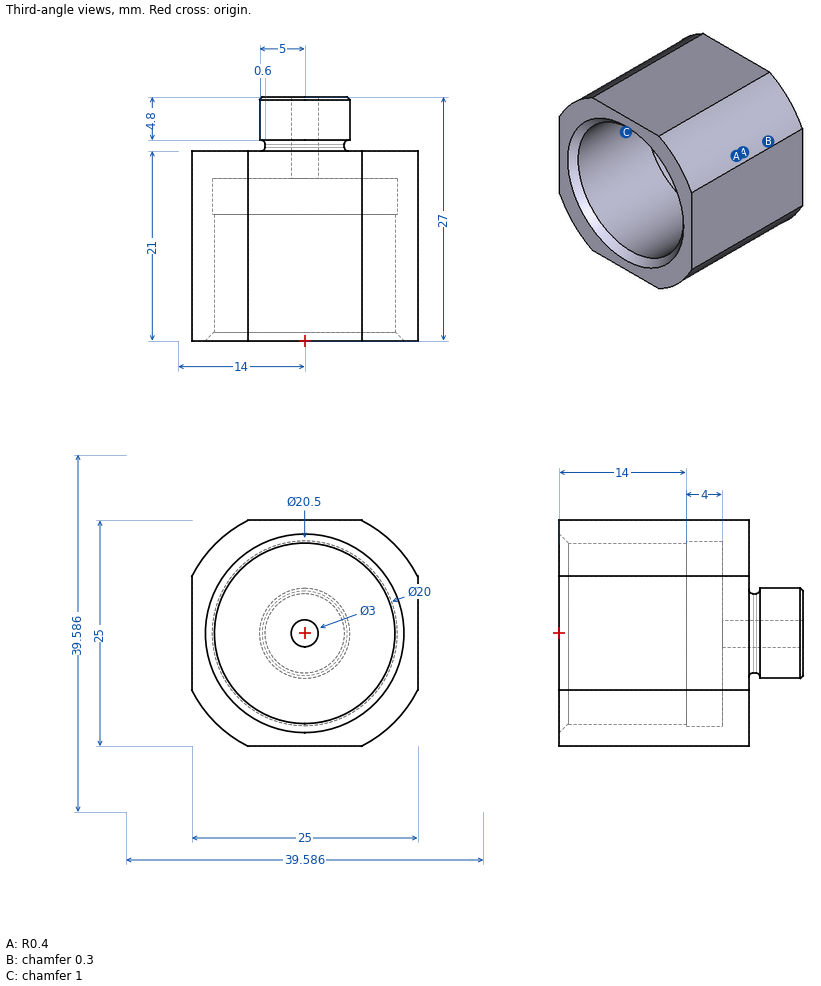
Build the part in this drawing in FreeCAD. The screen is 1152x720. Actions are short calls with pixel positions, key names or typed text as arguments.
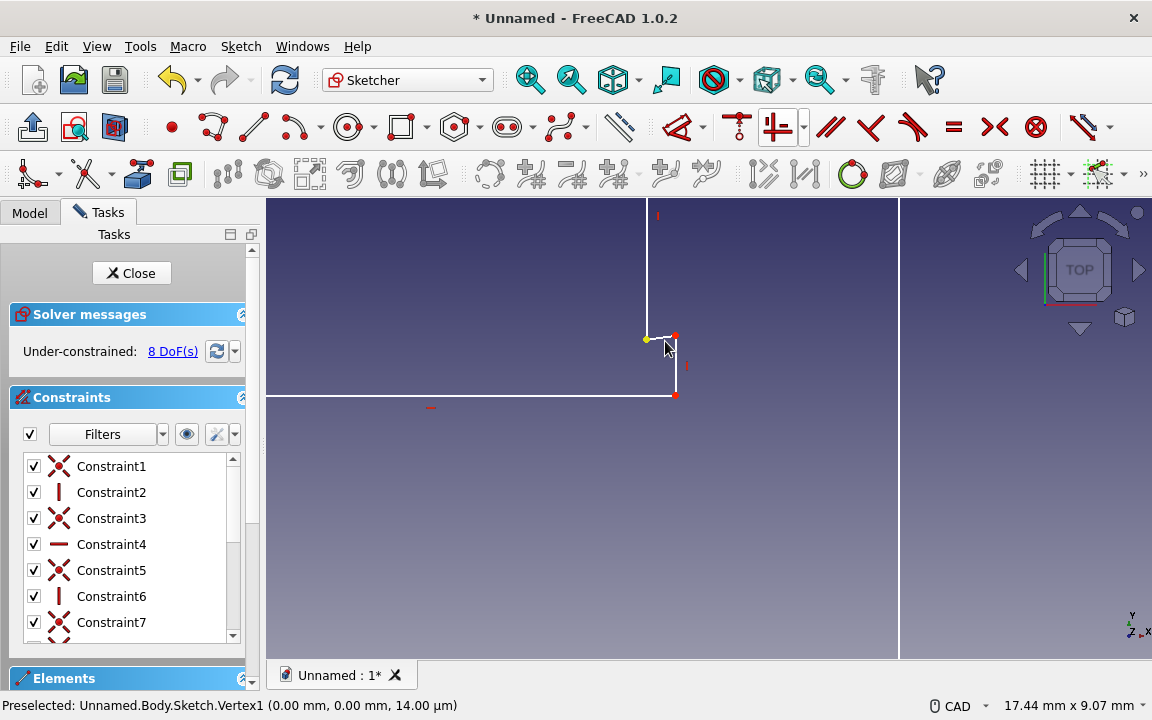
click(661, 338)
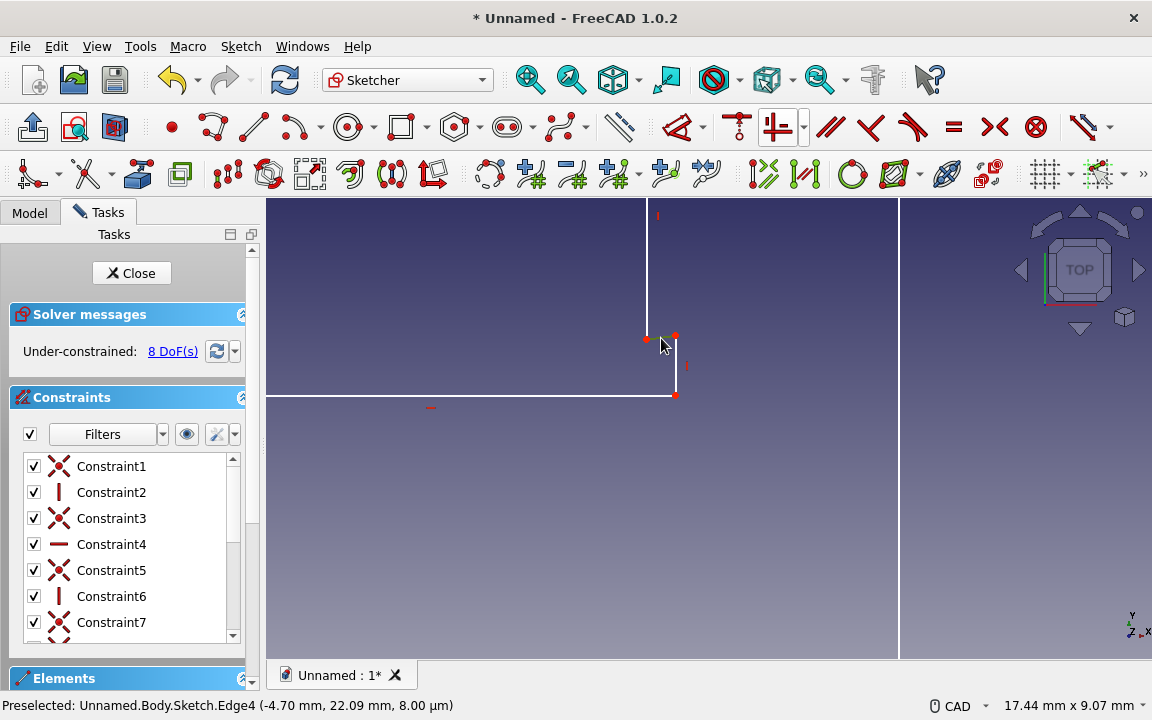
key(h)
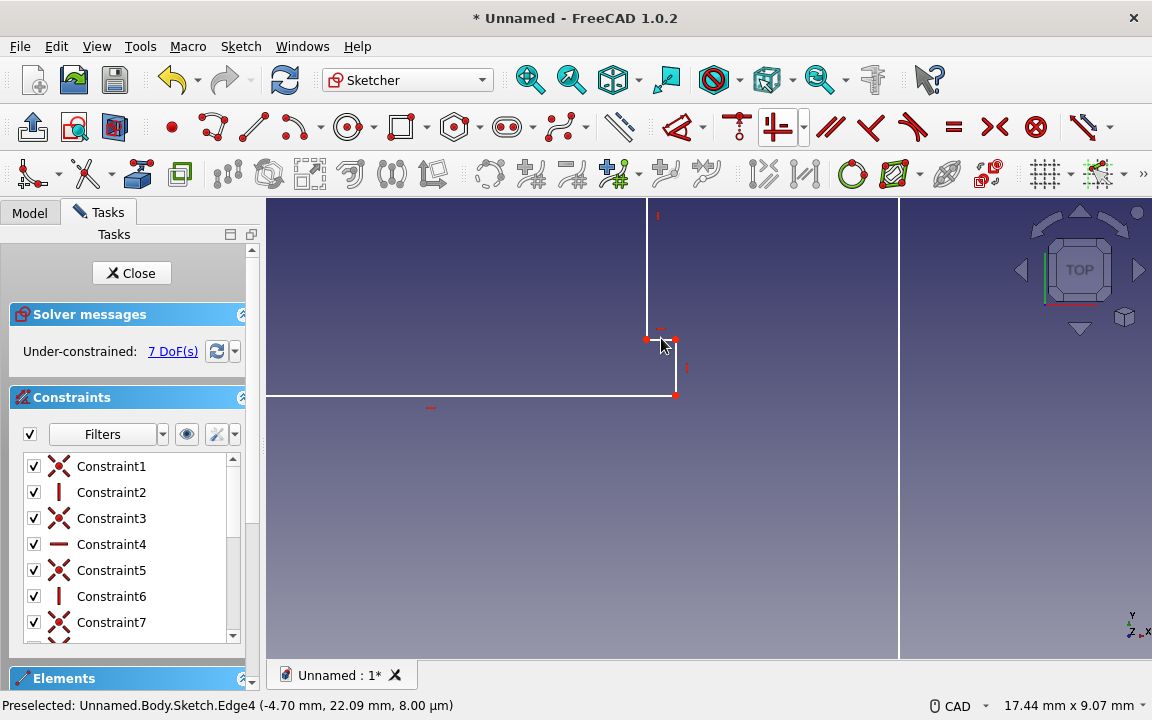
scroll(665, 341, down, 8)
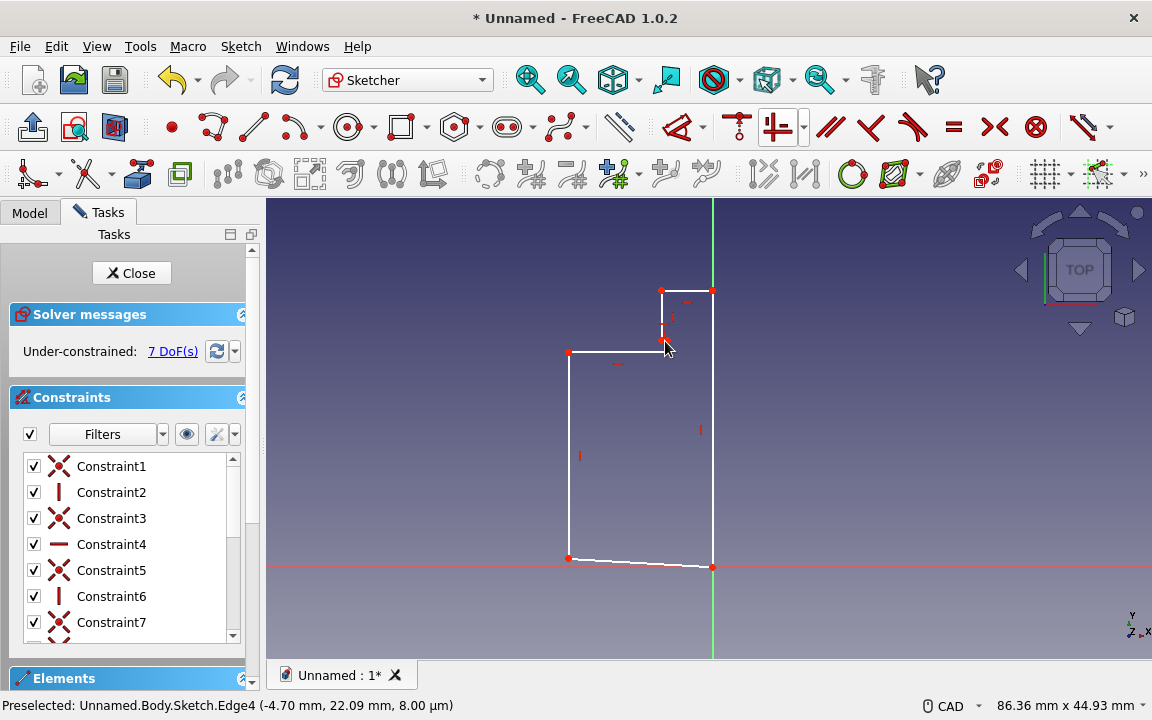
scroll(612, 561, up, 5)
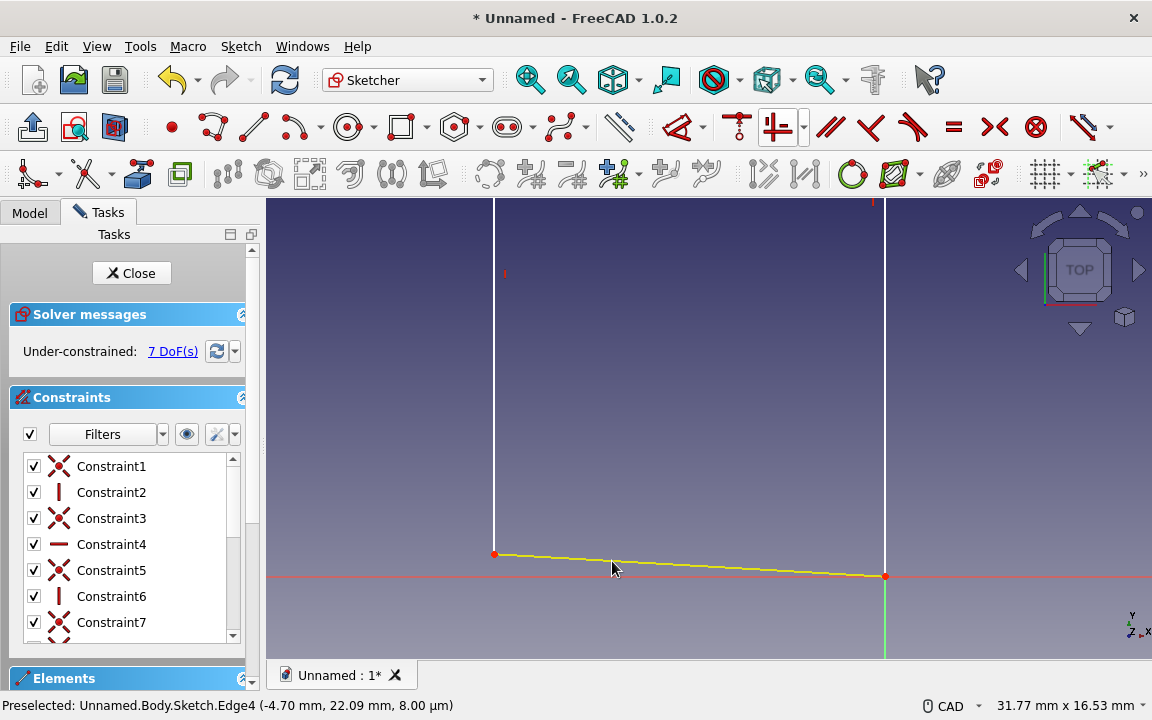
click(612, 561)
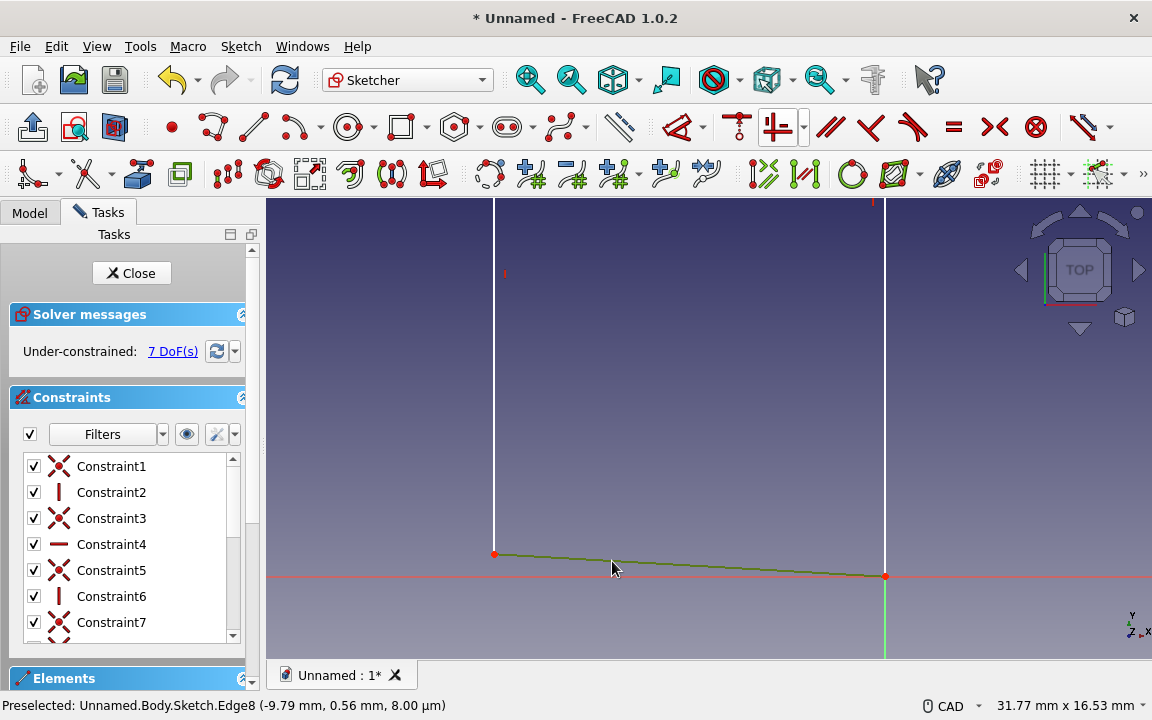
click(804, 128)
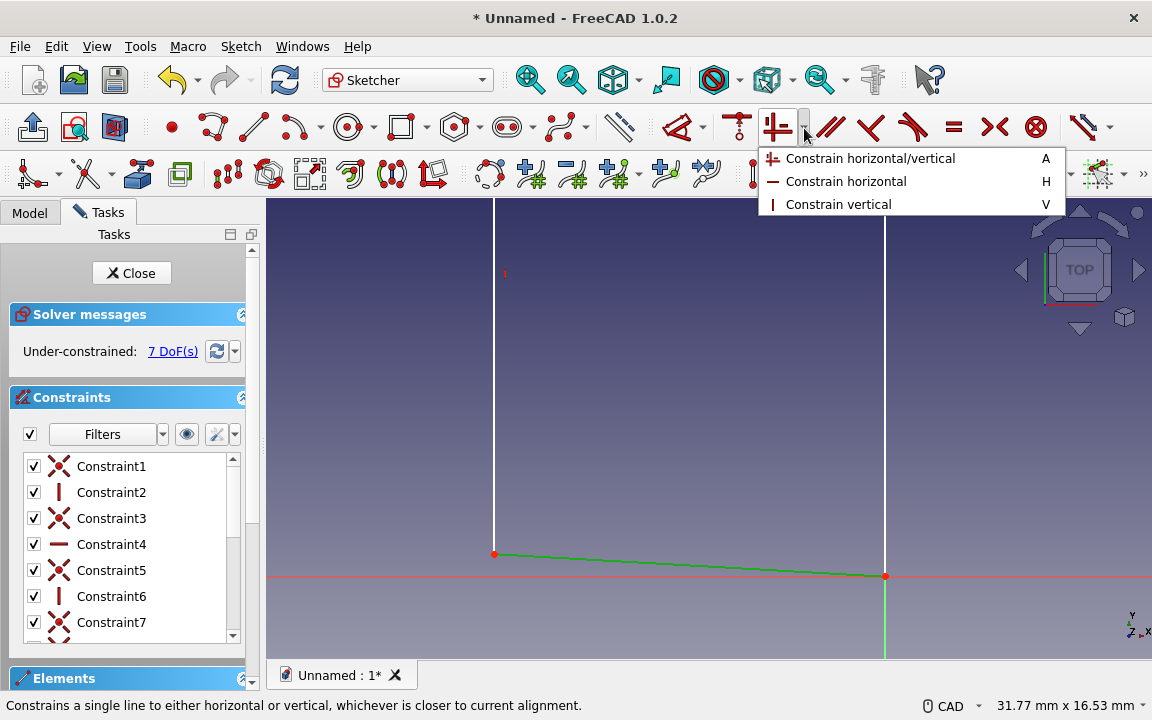
click(912, 182)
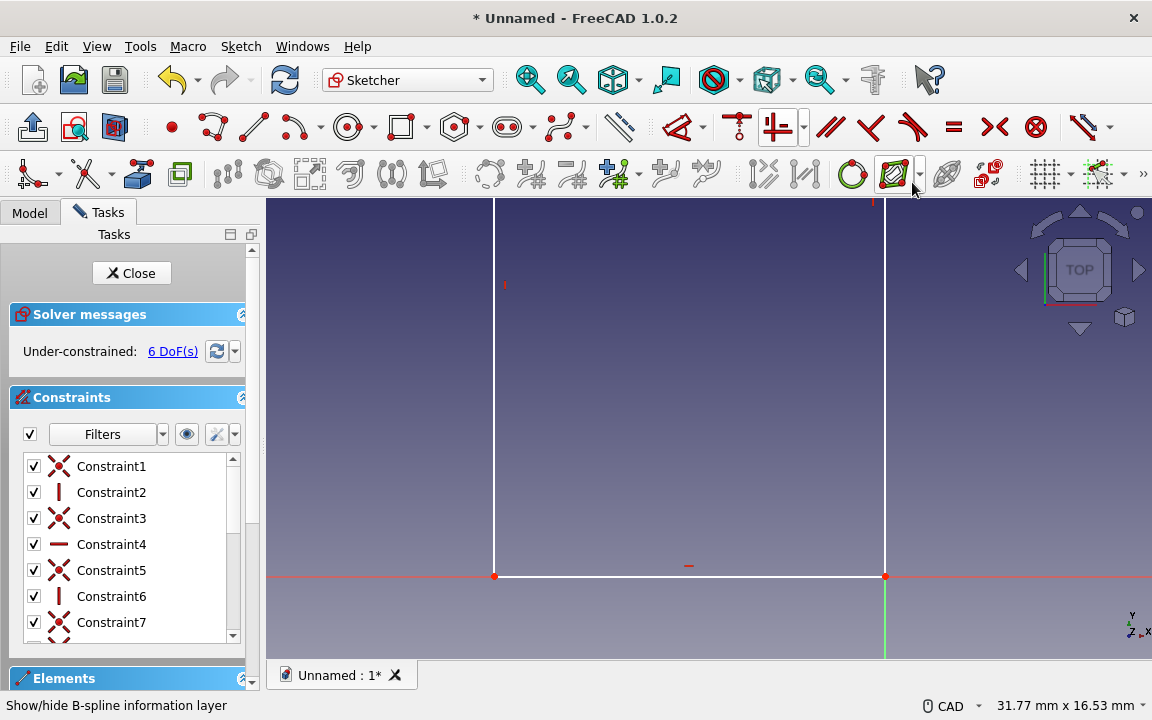
click(676, 128)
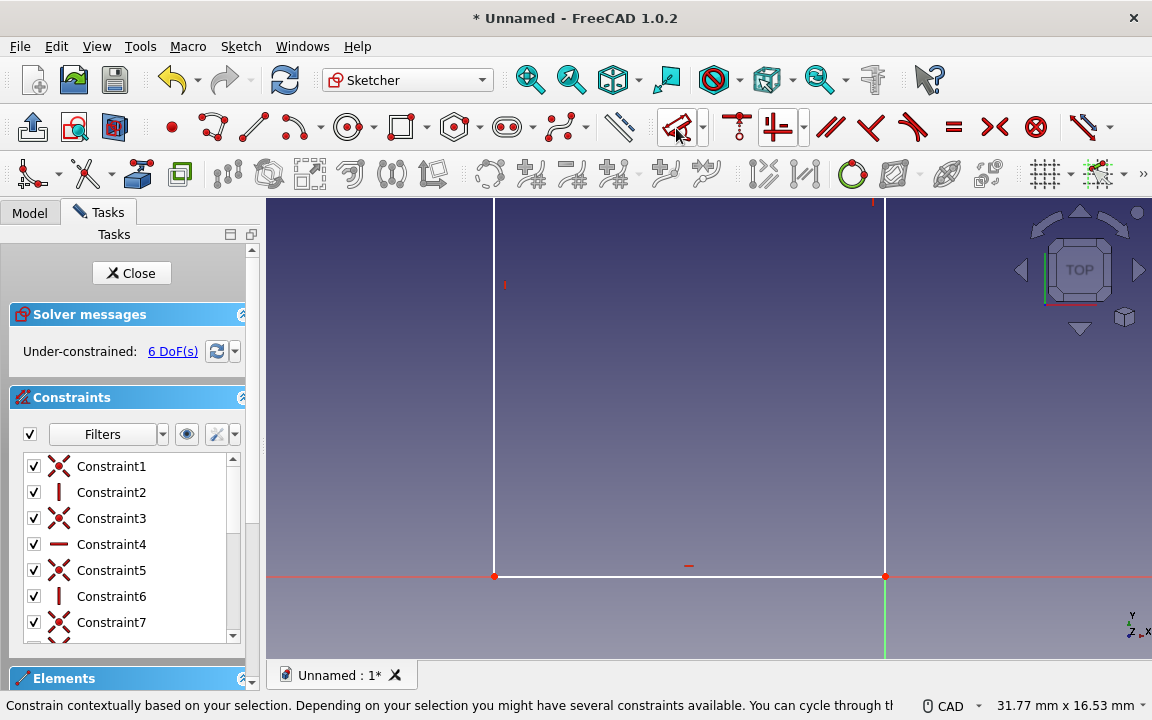
scroll(612, 561, down, 5)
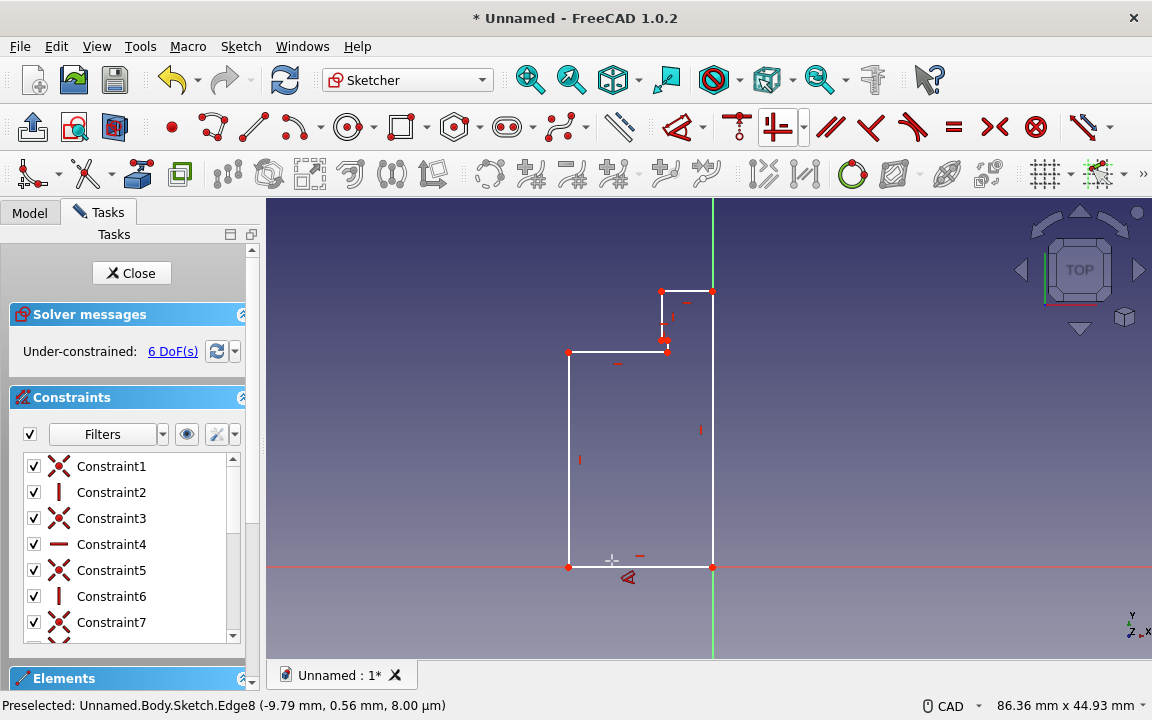
click(697, 291)
click(687, 257)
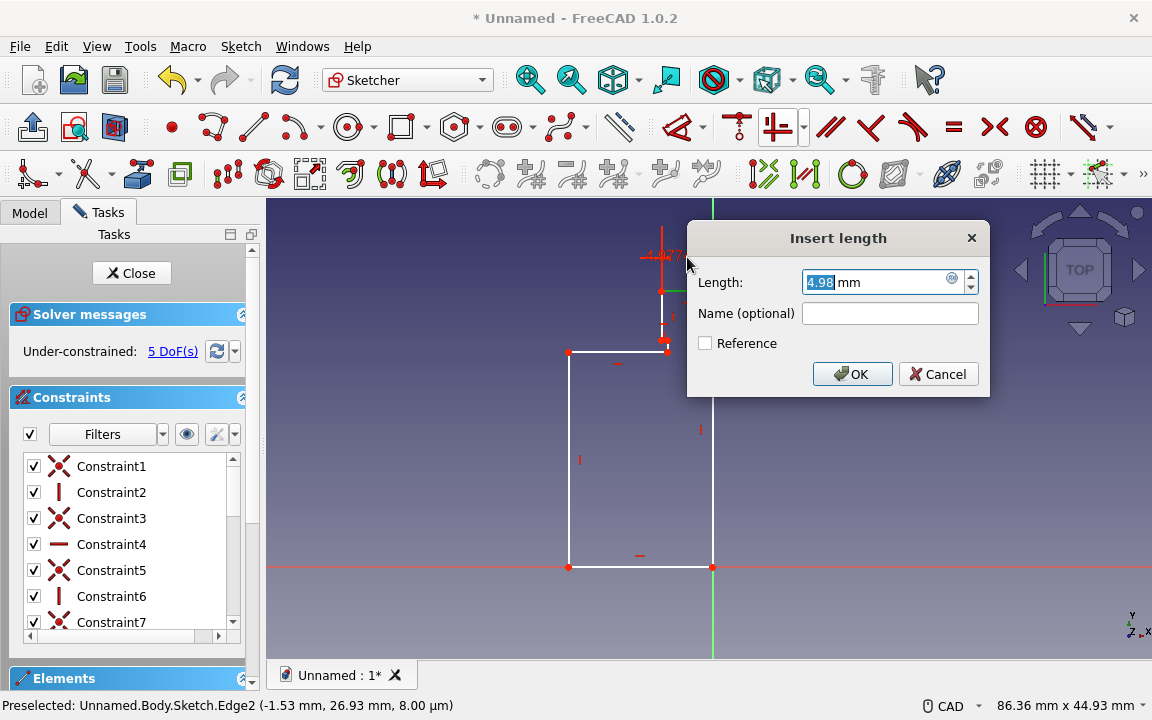
text(5)
key(Return)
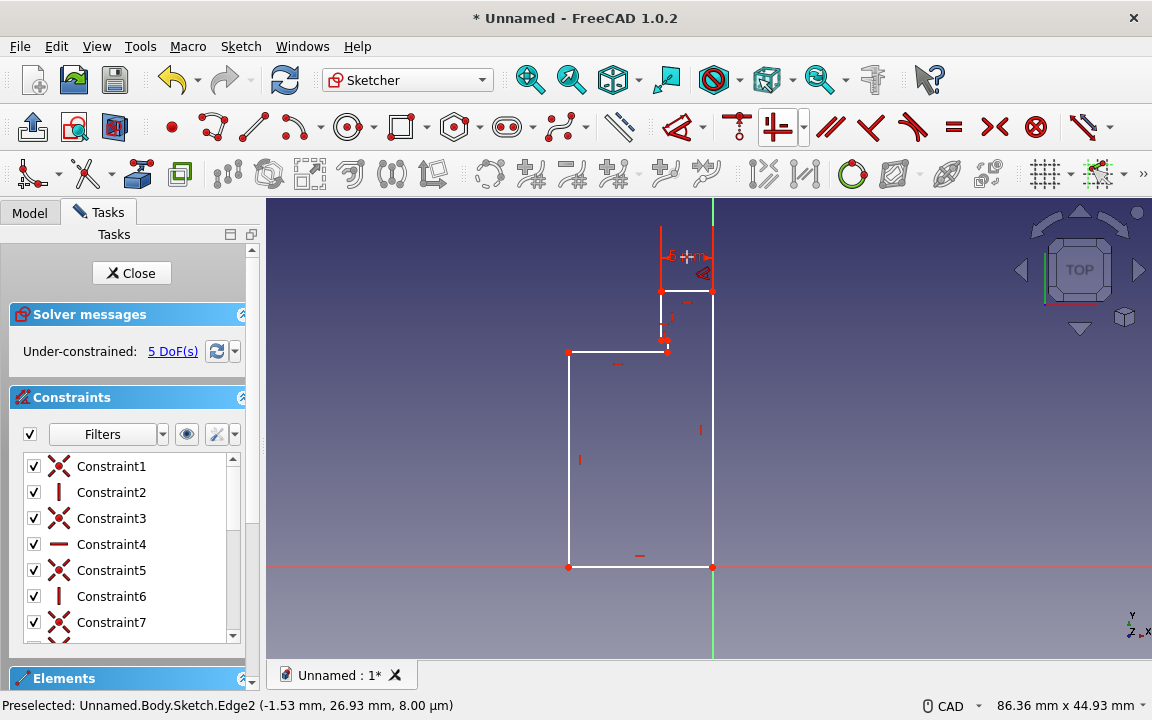
click(713, 484)
click(747, 429)